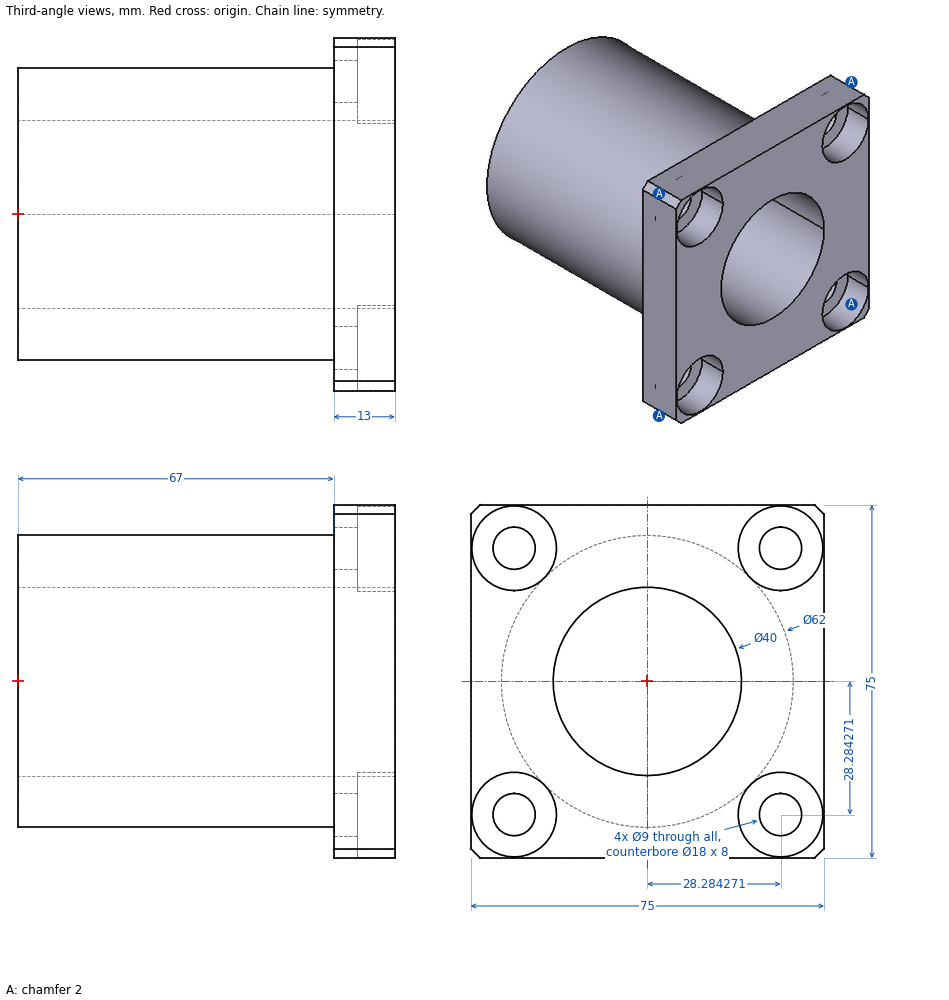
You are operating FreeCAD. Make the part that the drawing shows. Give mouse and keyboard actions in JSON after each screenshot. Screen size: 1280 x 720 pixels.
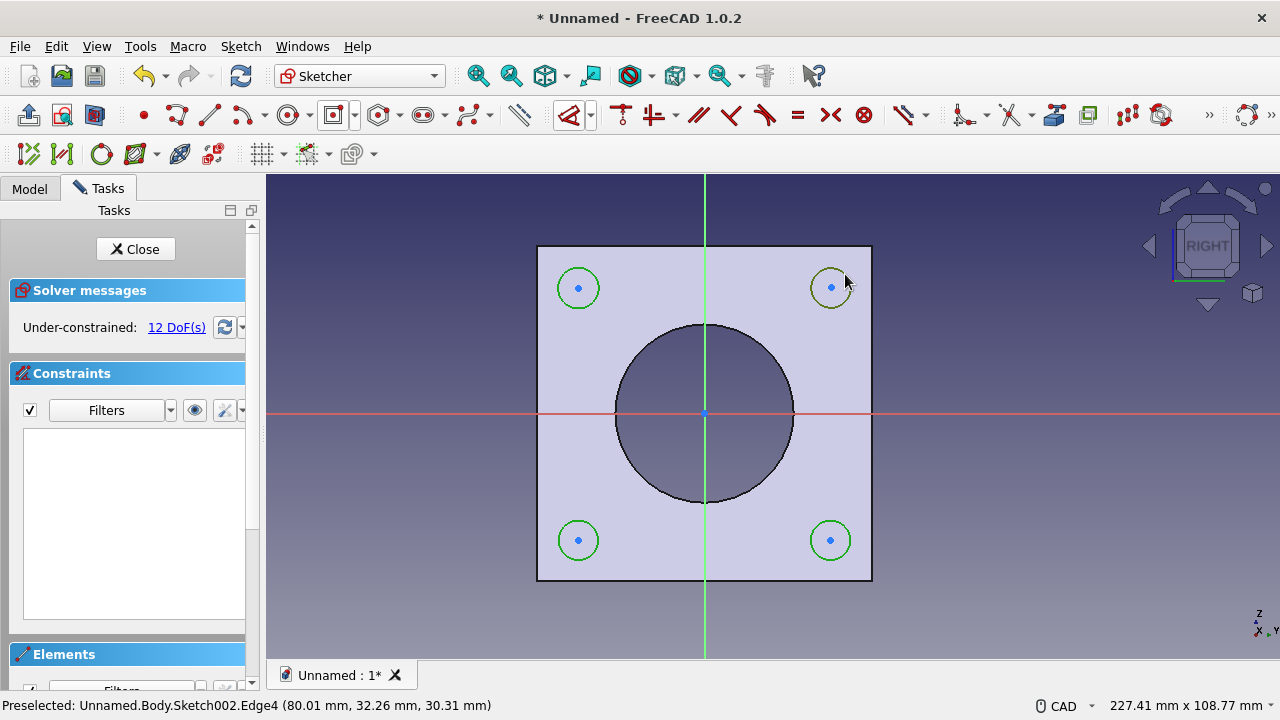
{"action": "left_click", "coordinate": [798, 116]}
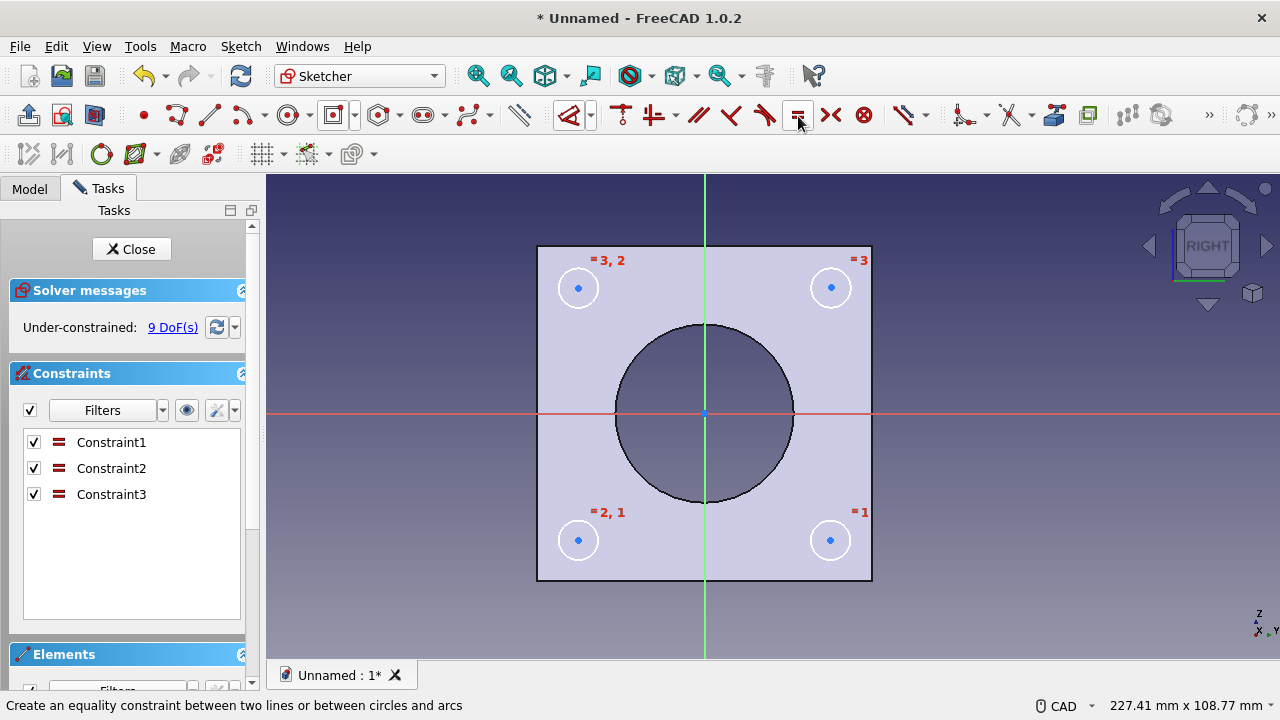
{"action": "left_click", "coordinate": [831, 540]}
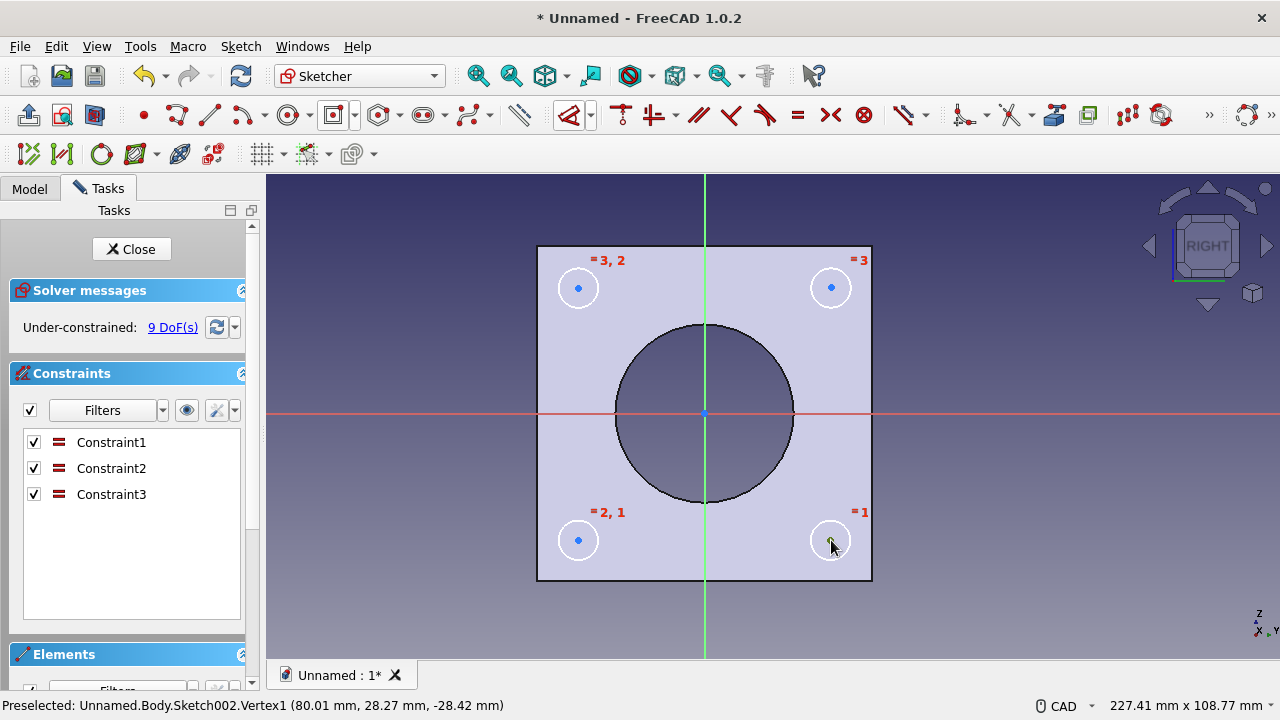
{"action": "left_click", "coordinate": [578, 540]}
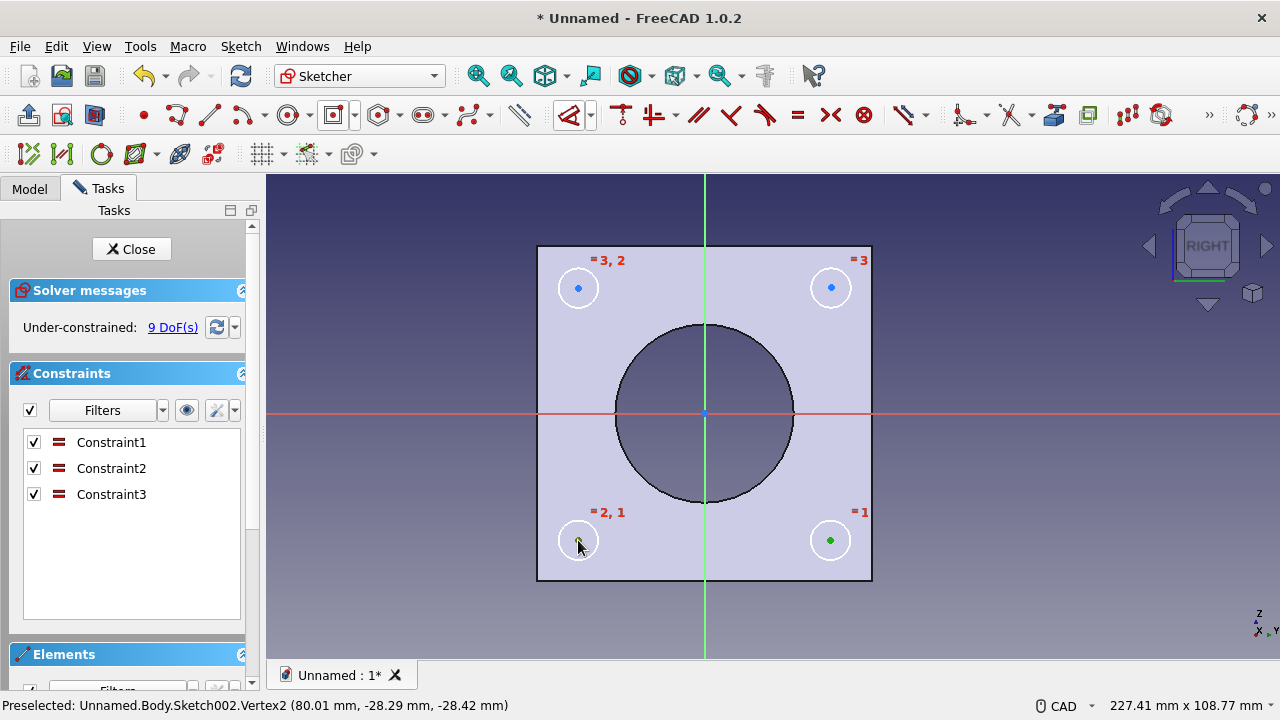
{"action": "left_click", "coordinate": [705, 600]}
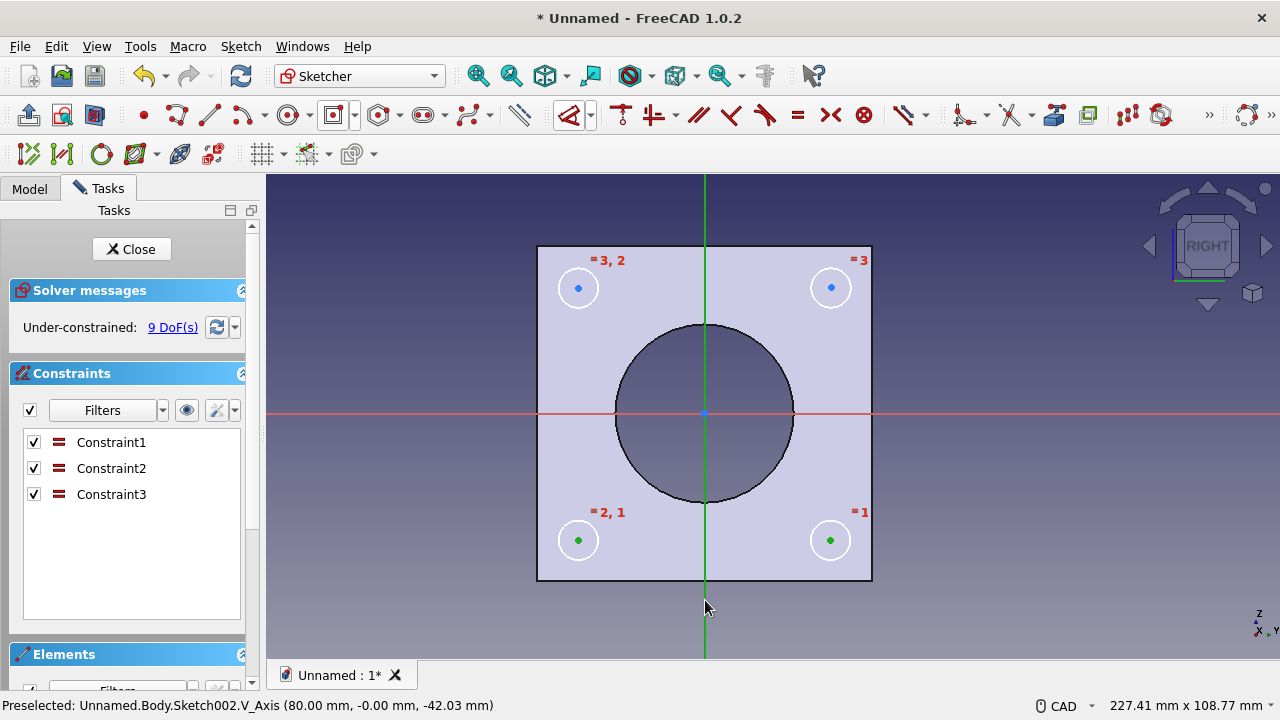
{"action": "left_click", "coordinate": [831, 116]}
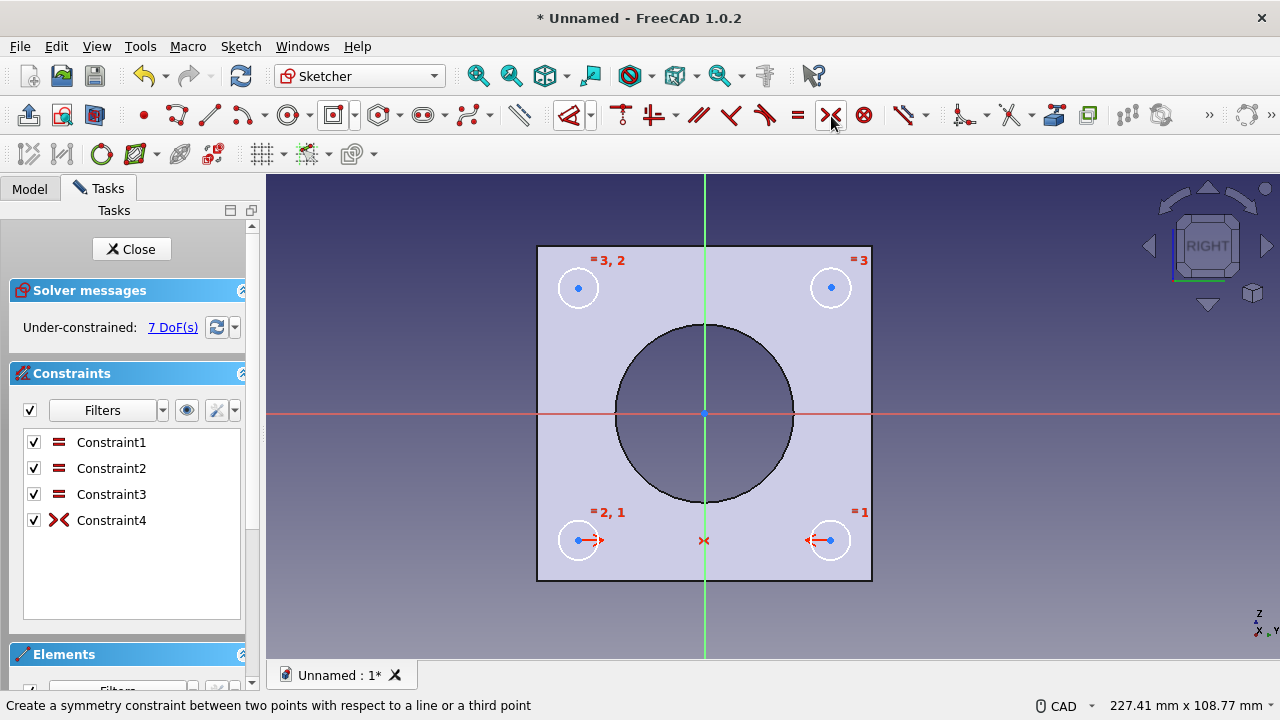
{"action": "left_click", "coordinate": [578, 540]}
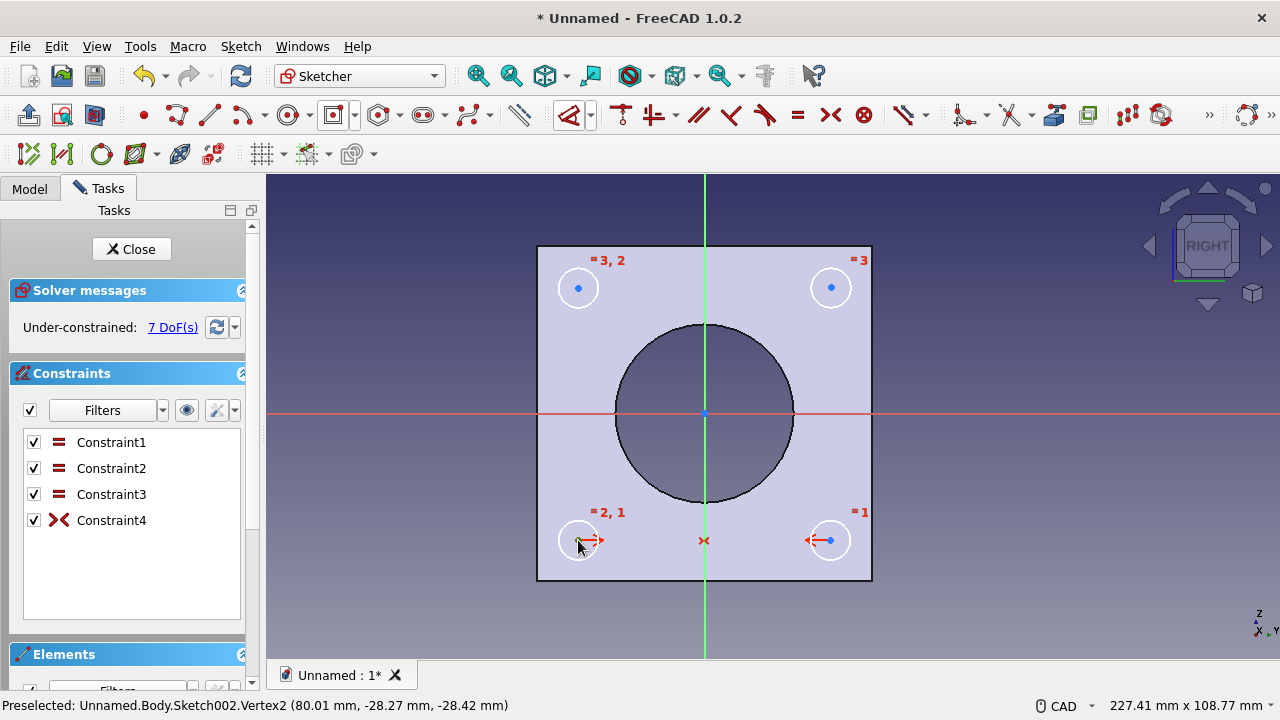
{"action": "left_click", "coordinate": [578, 288]}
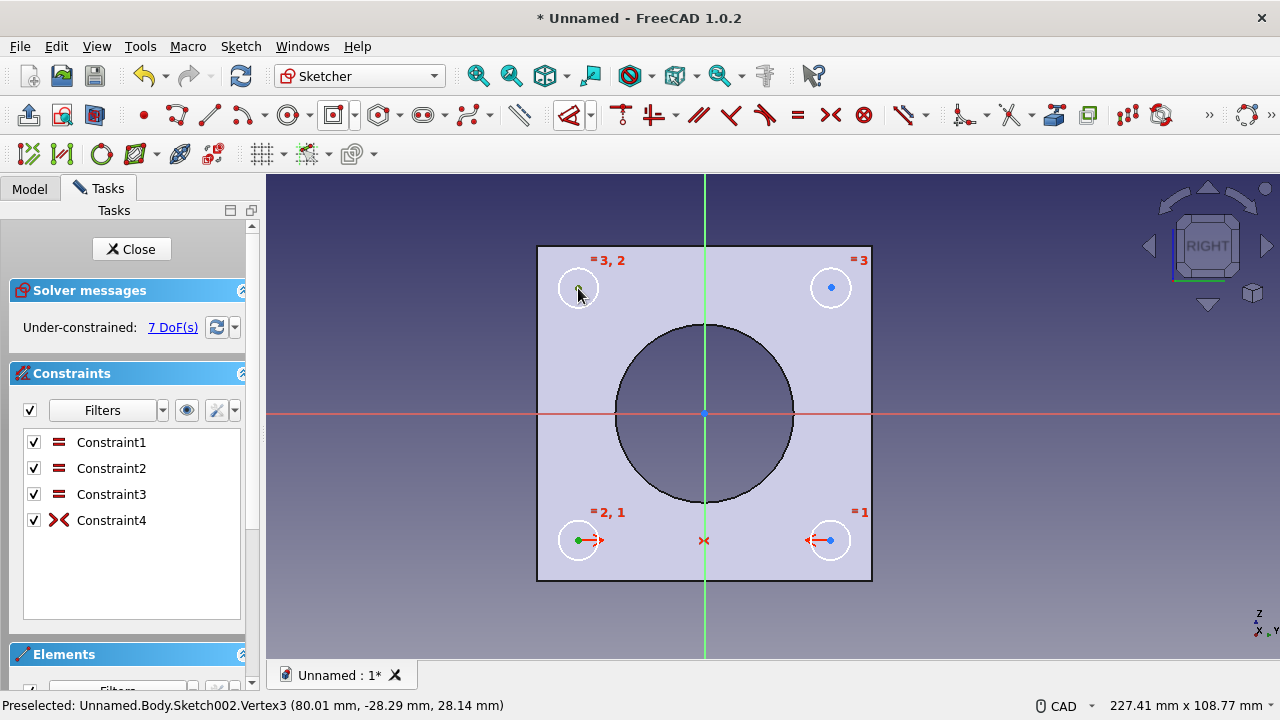
{"action": "left_click", "coordinate": [353, 414]}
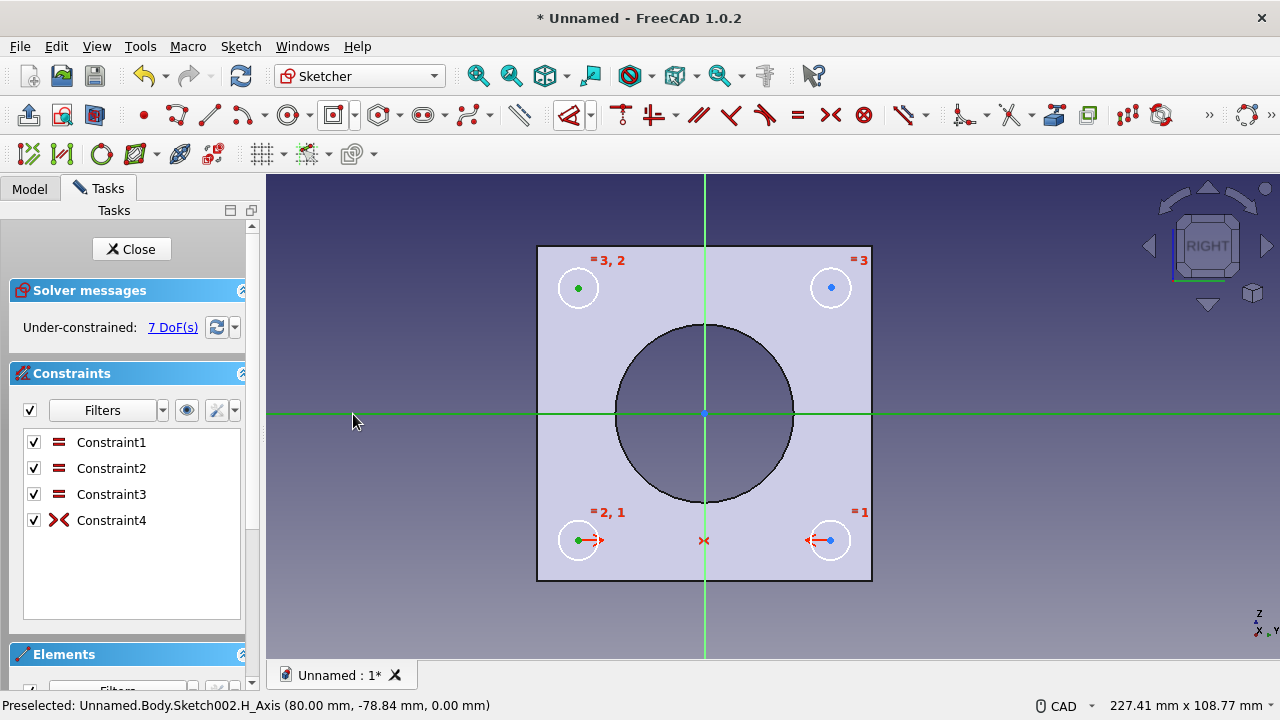
{"action": "left_click", "coordinate": [831, 116]}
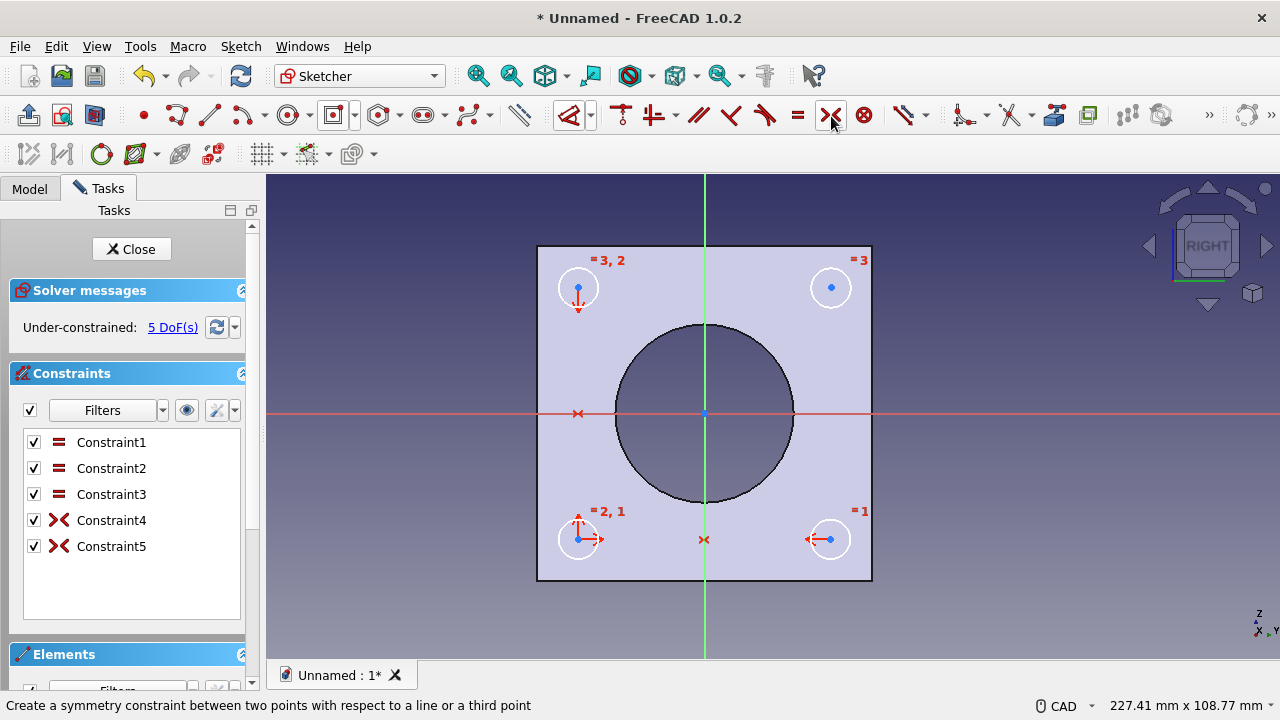
{"action": "left_click", "coordinate": [831, 539]}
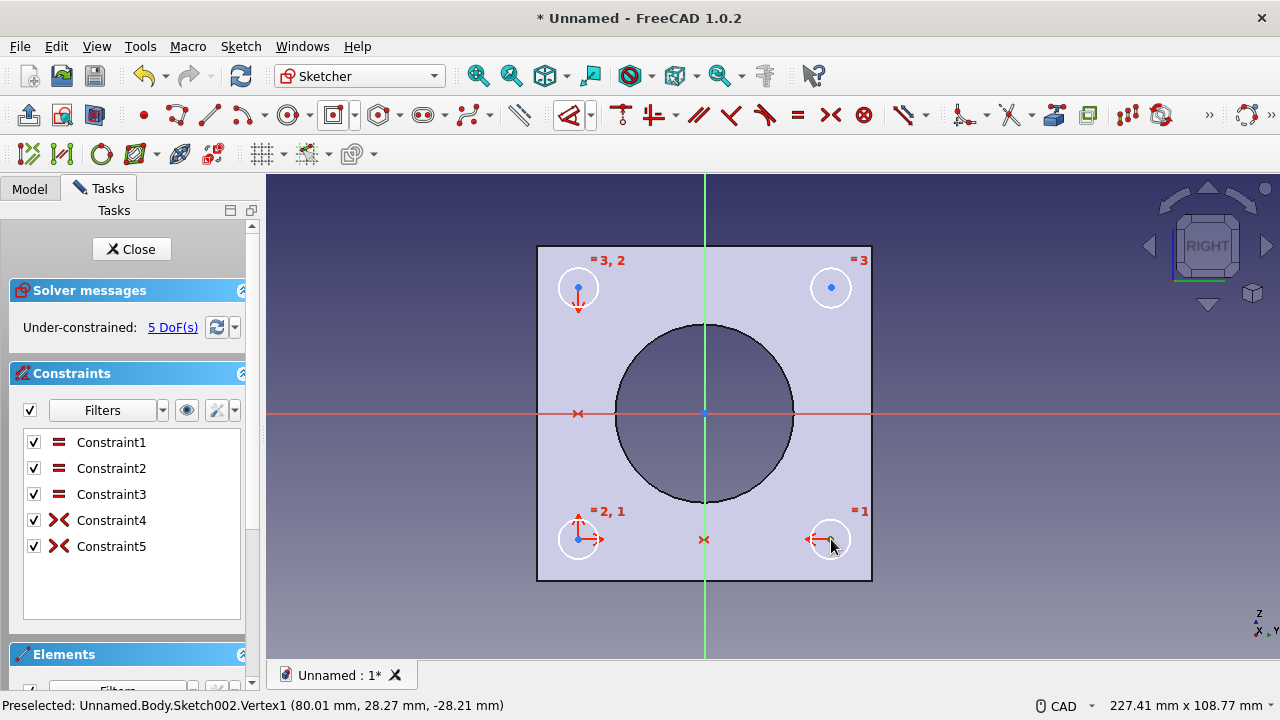
{"action": "left_click", "coordinate": [831, 288]}